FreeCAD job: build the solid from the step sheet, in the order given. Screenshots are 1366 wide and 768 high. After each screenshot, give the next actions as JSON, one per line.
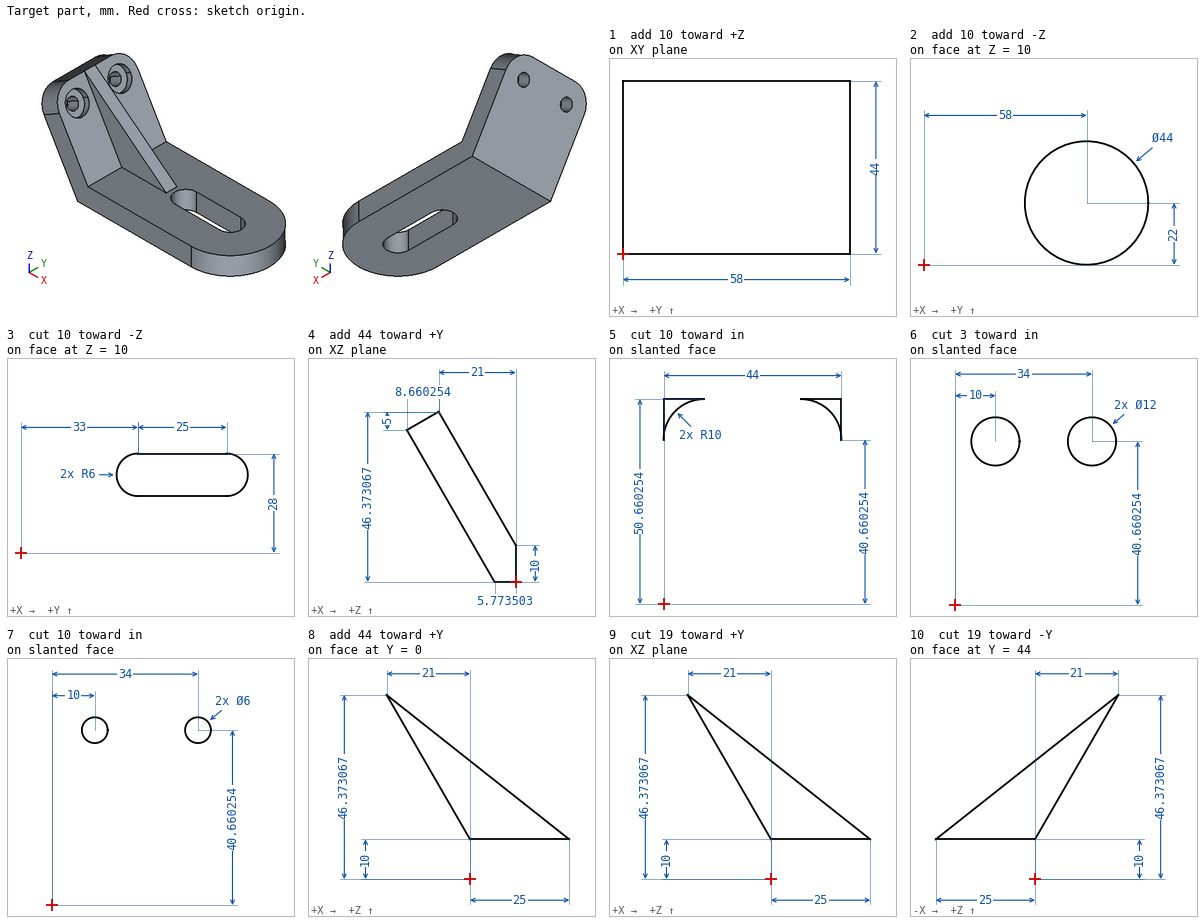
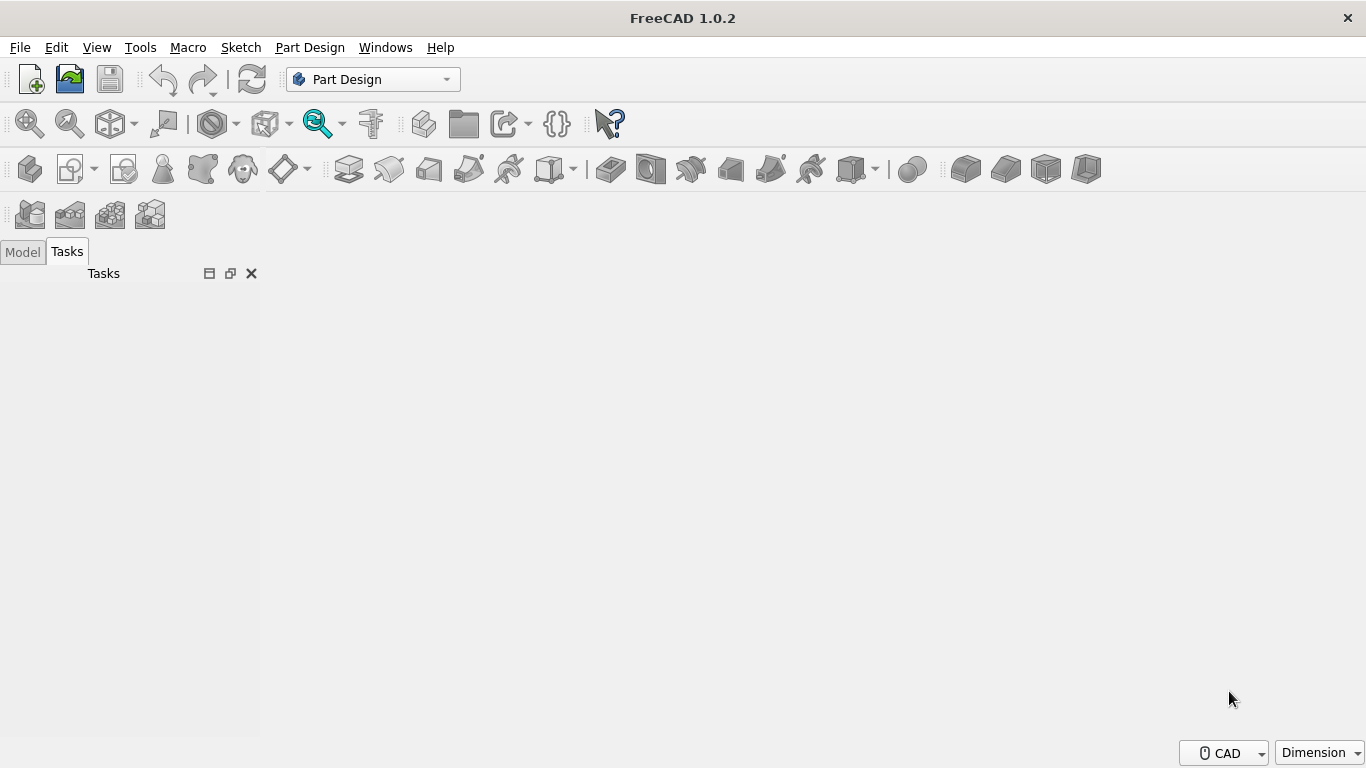
{"action": "left_click", "coordinate": [548, 124]}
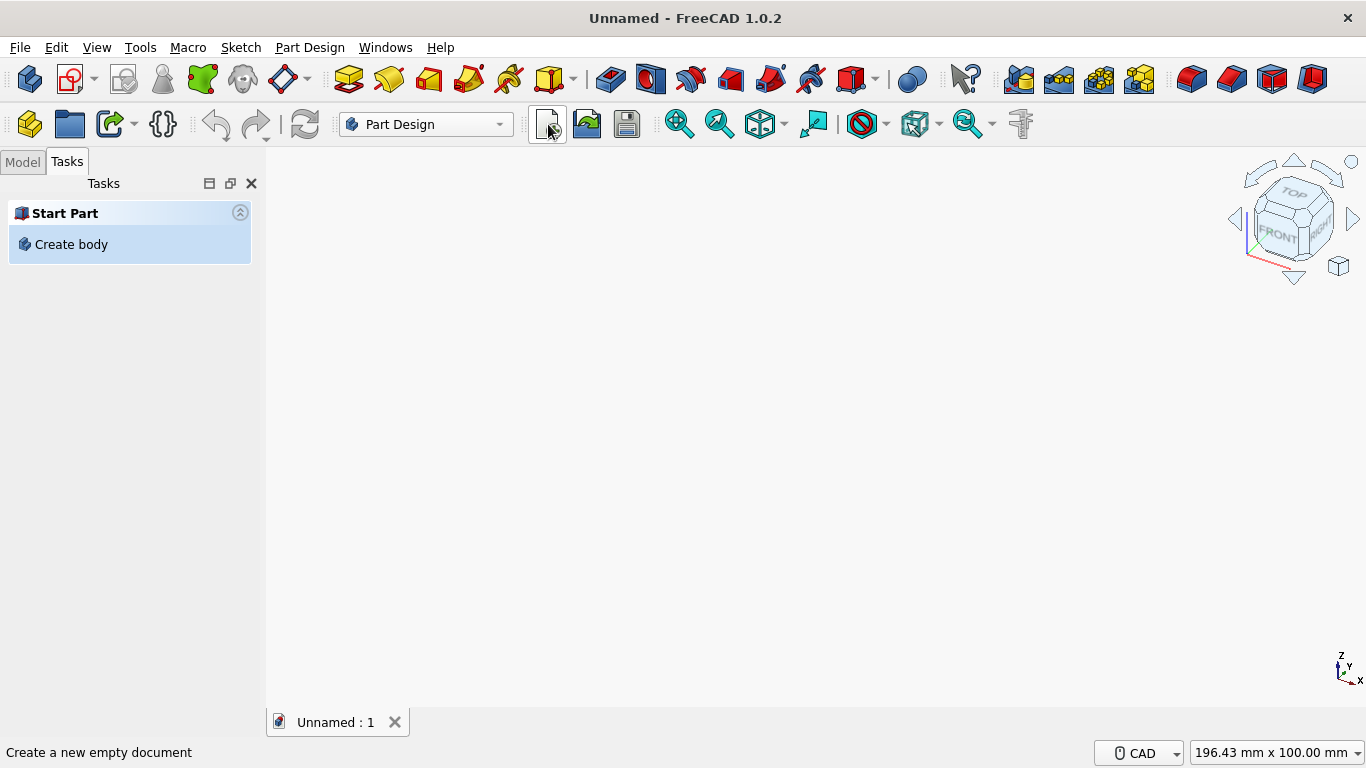
{"action": "left_click", "coordinate": [70, 80]}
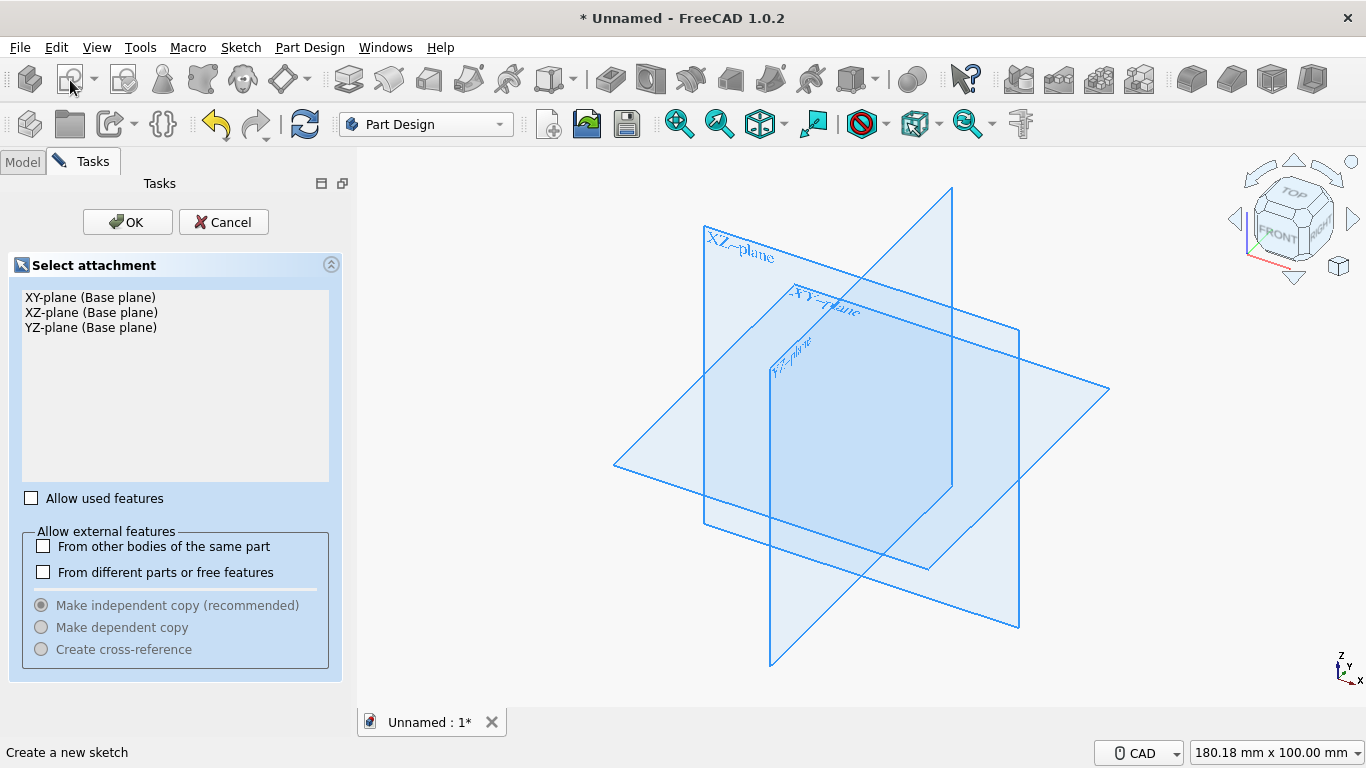
{"action": "left_click", "coordinate": [82, 298]}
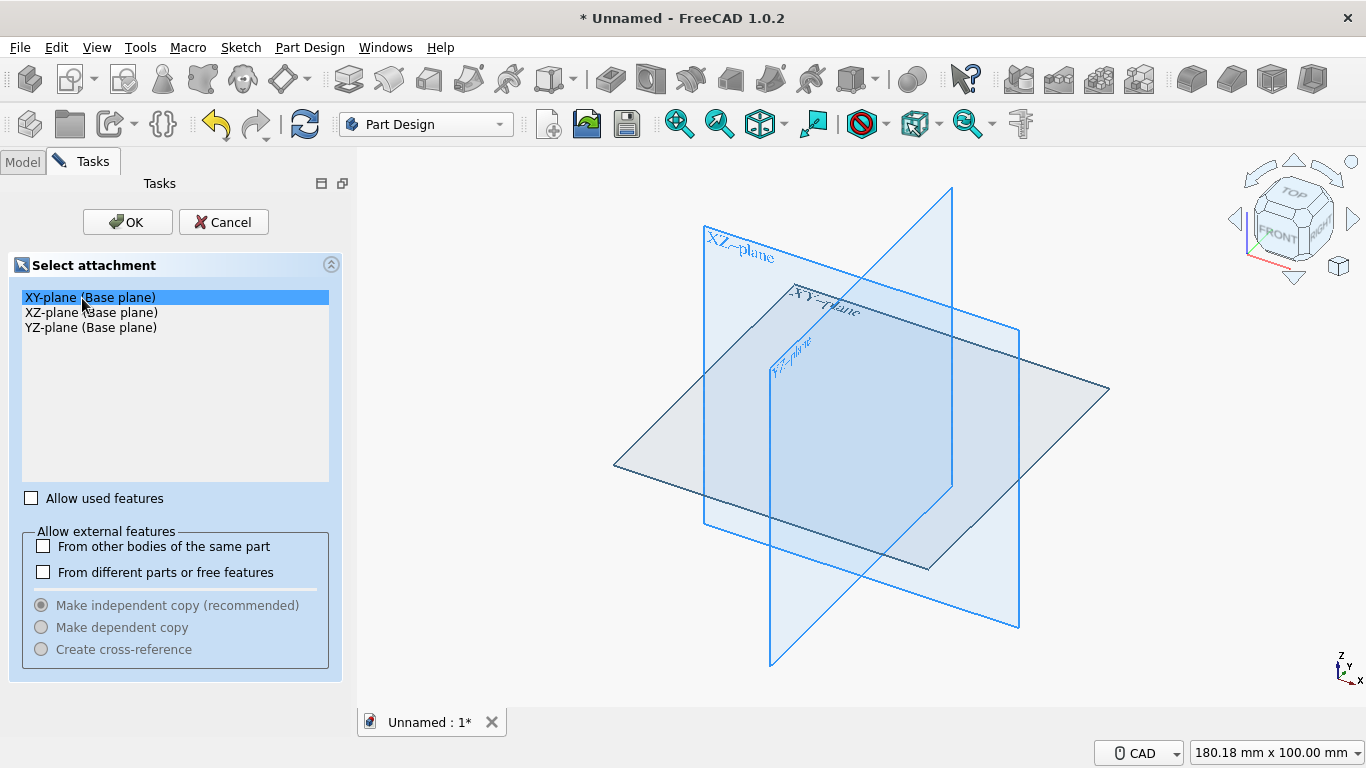
{"action": "left_click", "coordinate": [128, 222]}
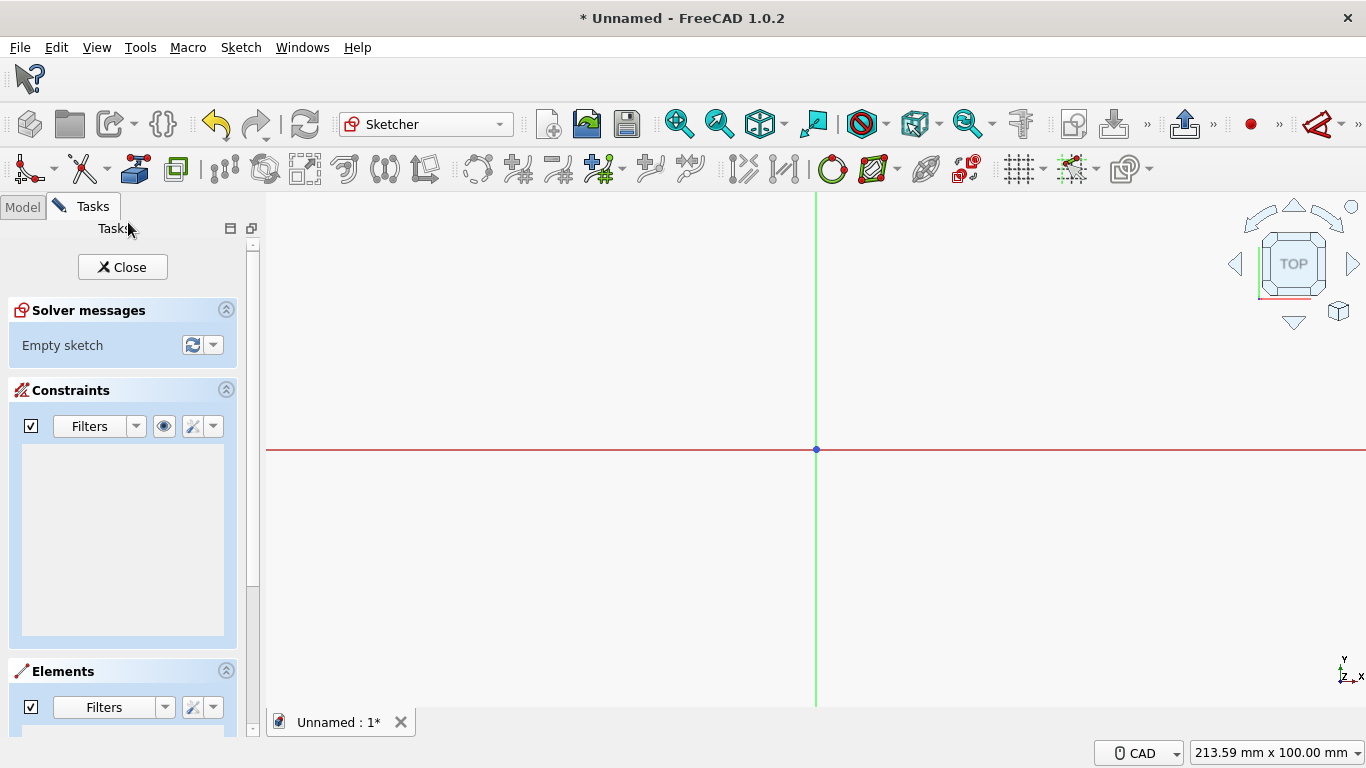
{"action": "scroll", "coordinate": [294, 679], "scroll_direction": "down", "scroll_amount": 1}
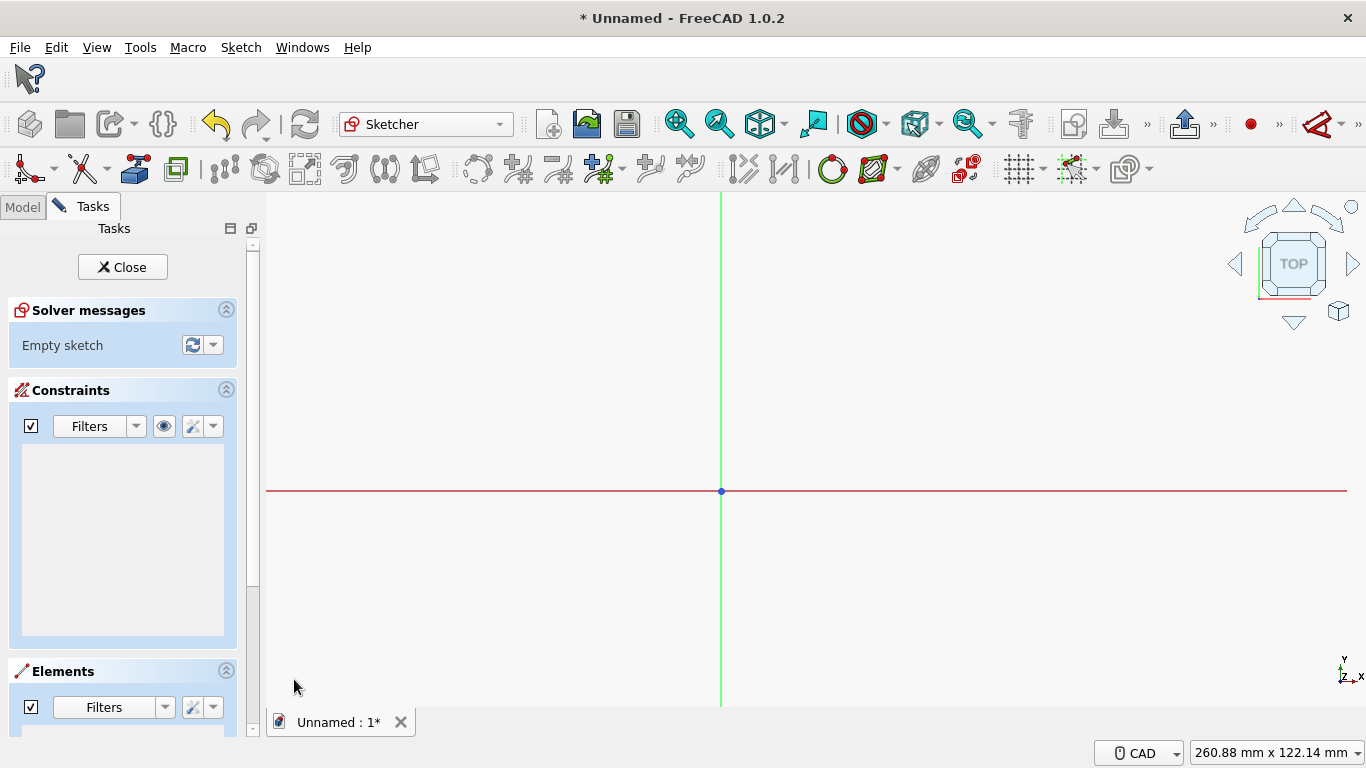
{"action": "scroll", "coordinate": [961, 336], "scroll_direction": "up", "scroll_amount": 3}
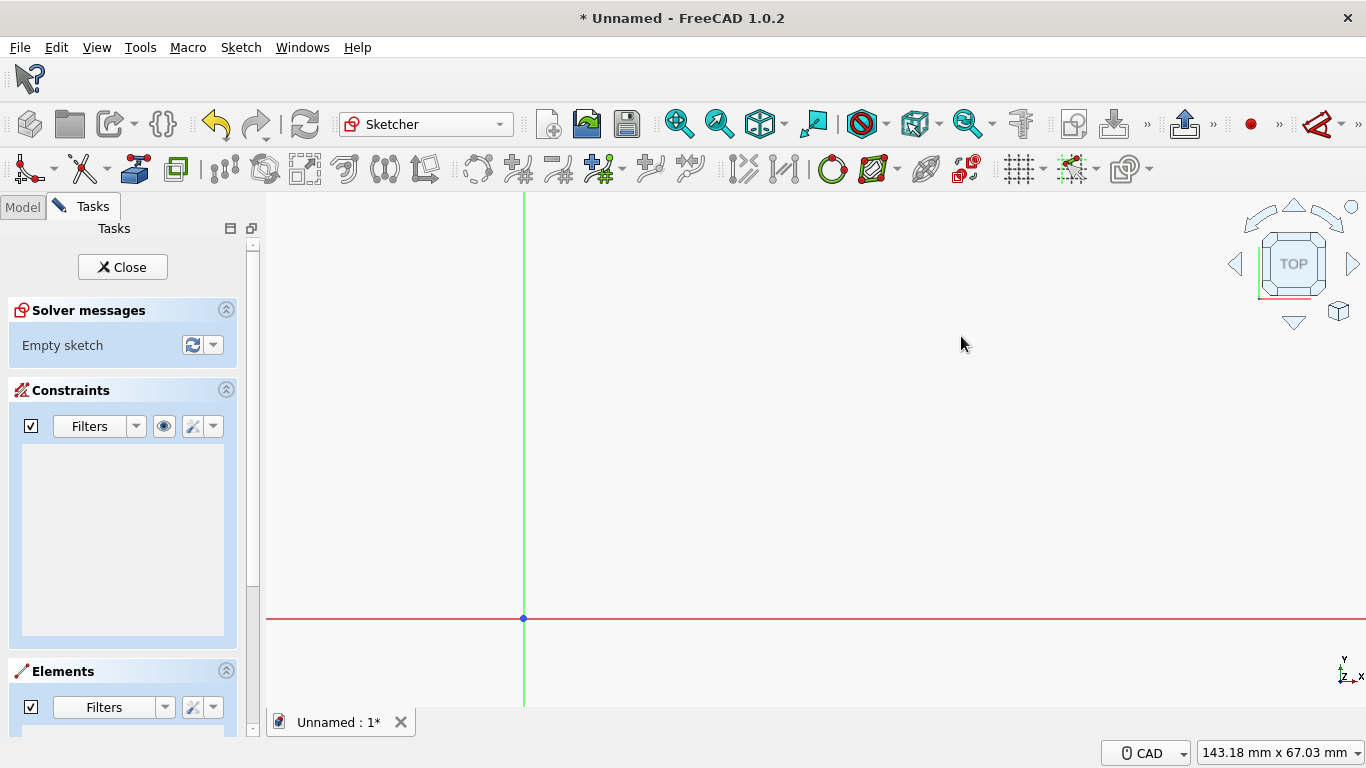
{"action": "key", "text": "g r"}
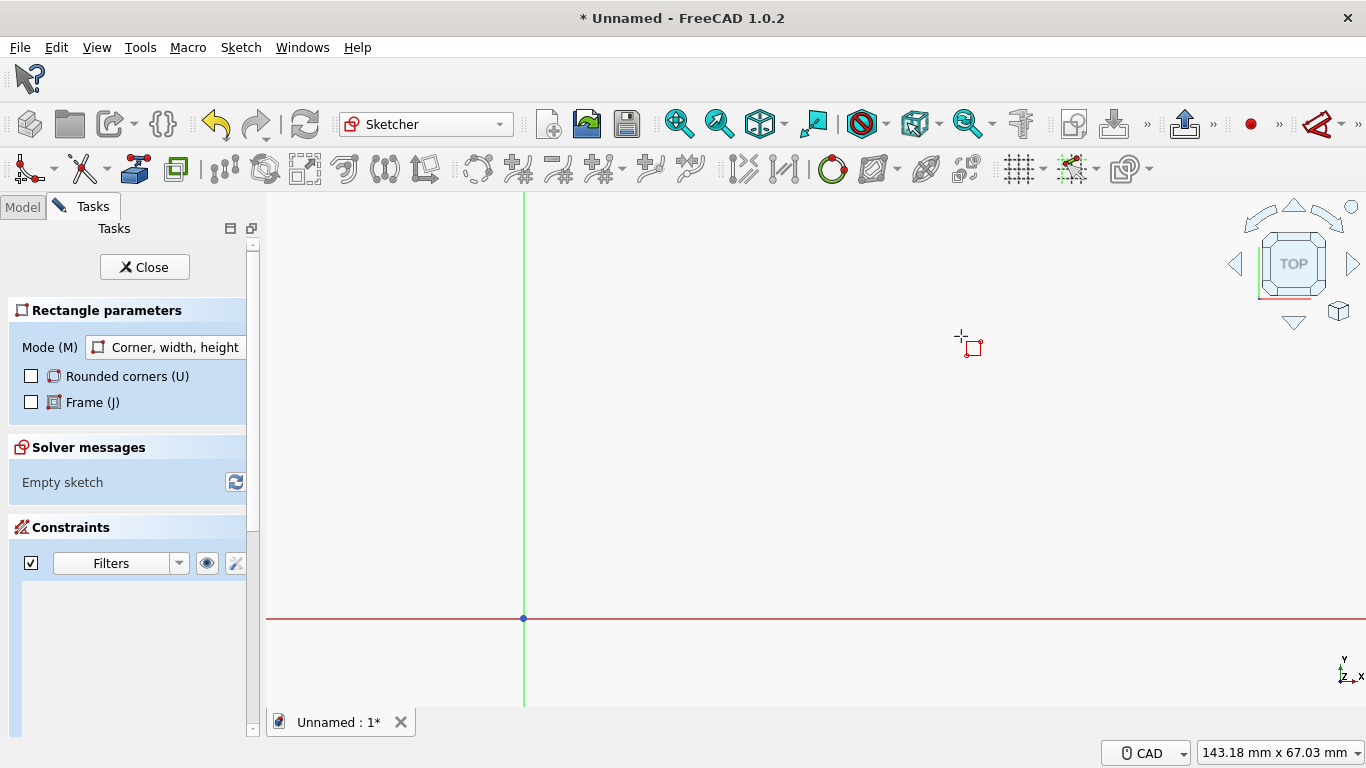
{"action": "left_click", "coordinate": [524, 619]}
{"action": "mouse_move", "coordinate": [969, 281]}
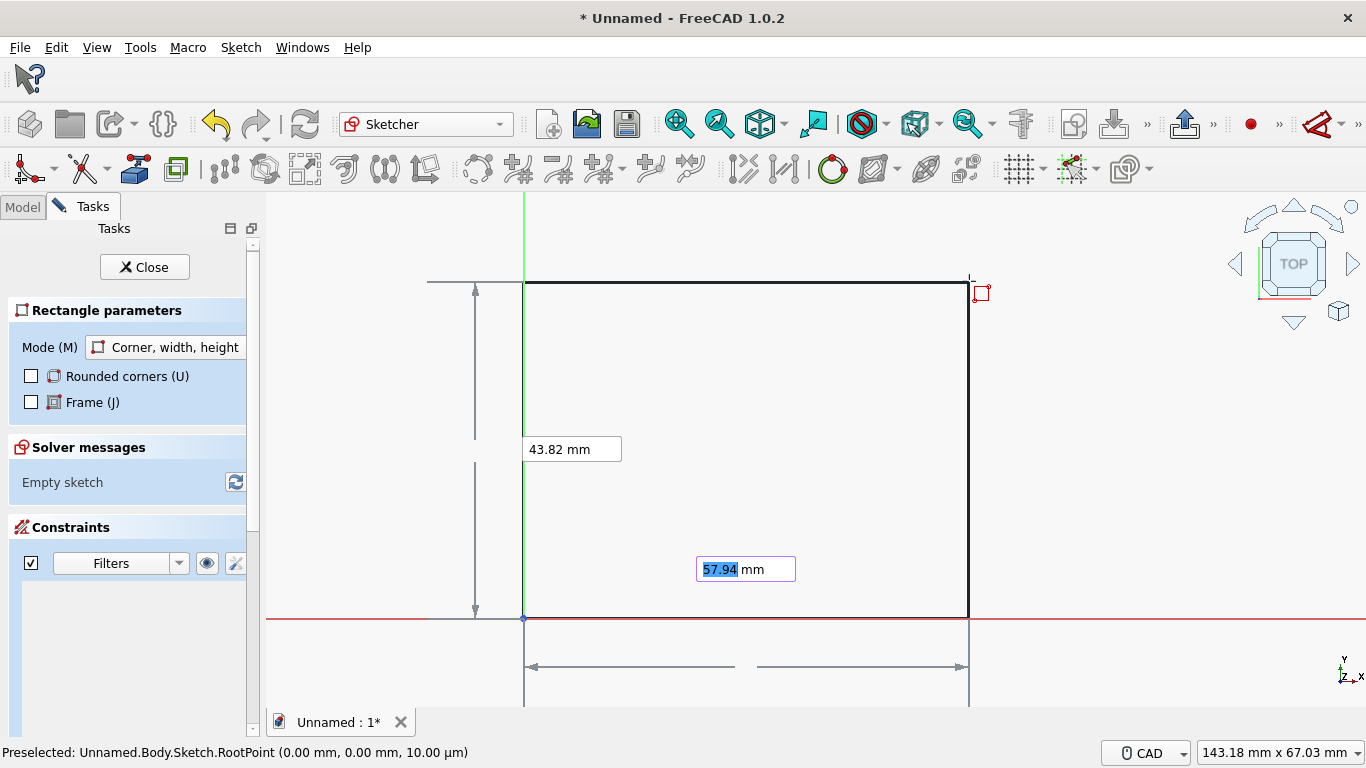
{"action": "type", "text": "58"}
{"action": "key", "text": "Tab"}
{"action": "type", "text": "44"}
{"action": "key", "text": "Return"}
{"action": "key", "text": "Escape"}